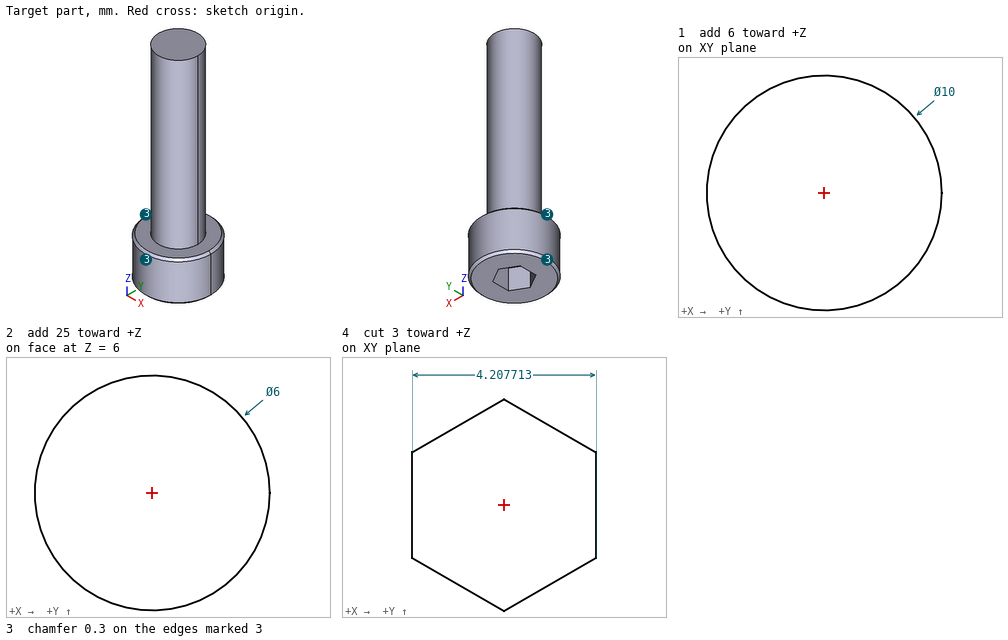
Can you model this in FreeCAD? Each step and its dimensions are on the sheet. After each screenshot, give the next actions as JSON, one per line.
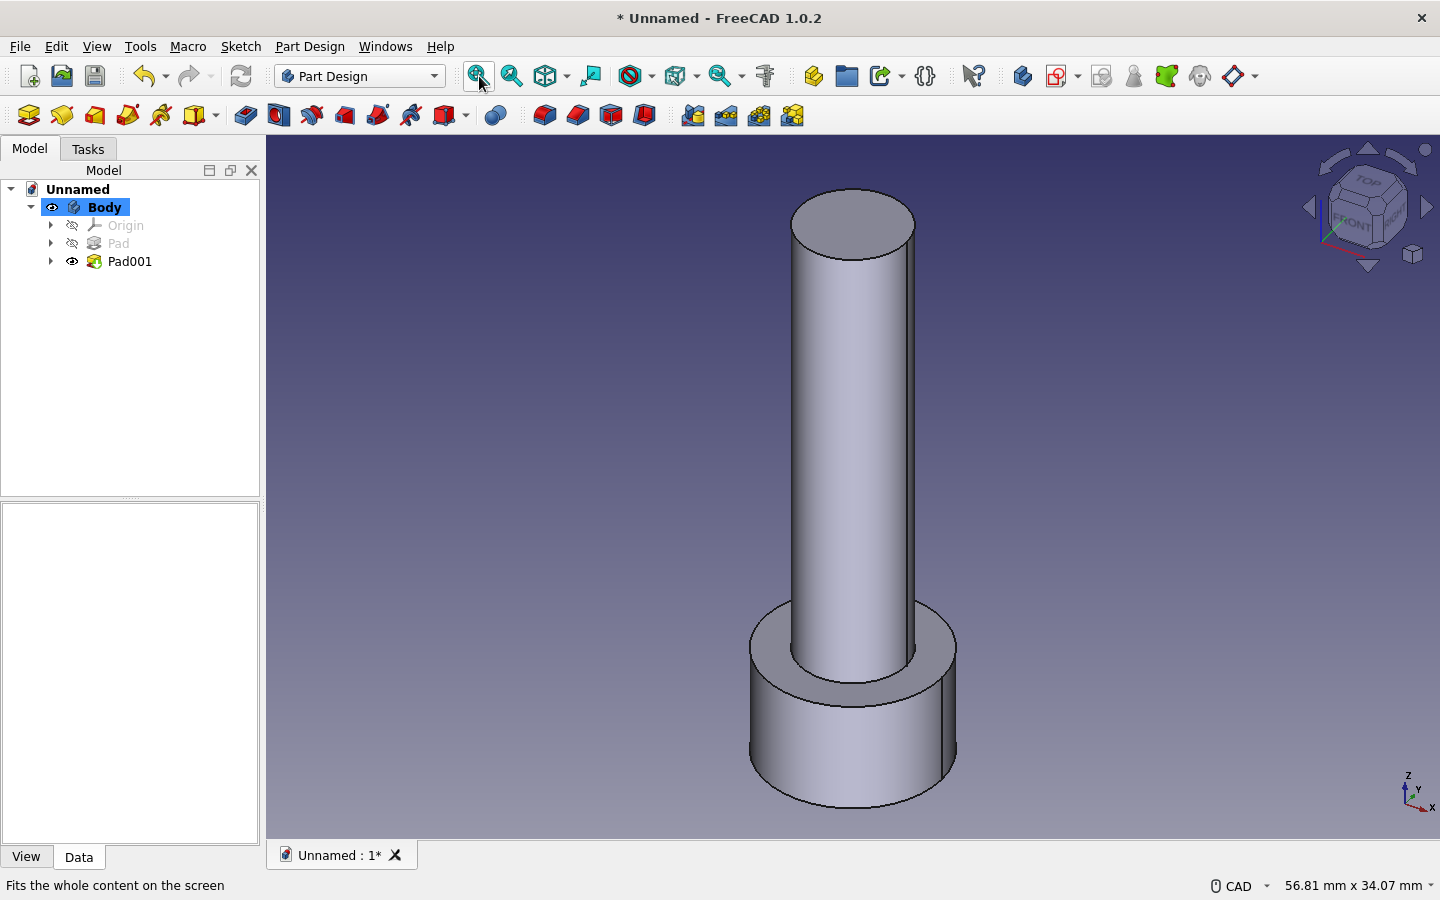
{"action": "left_click", "coordinate": [750, 653]}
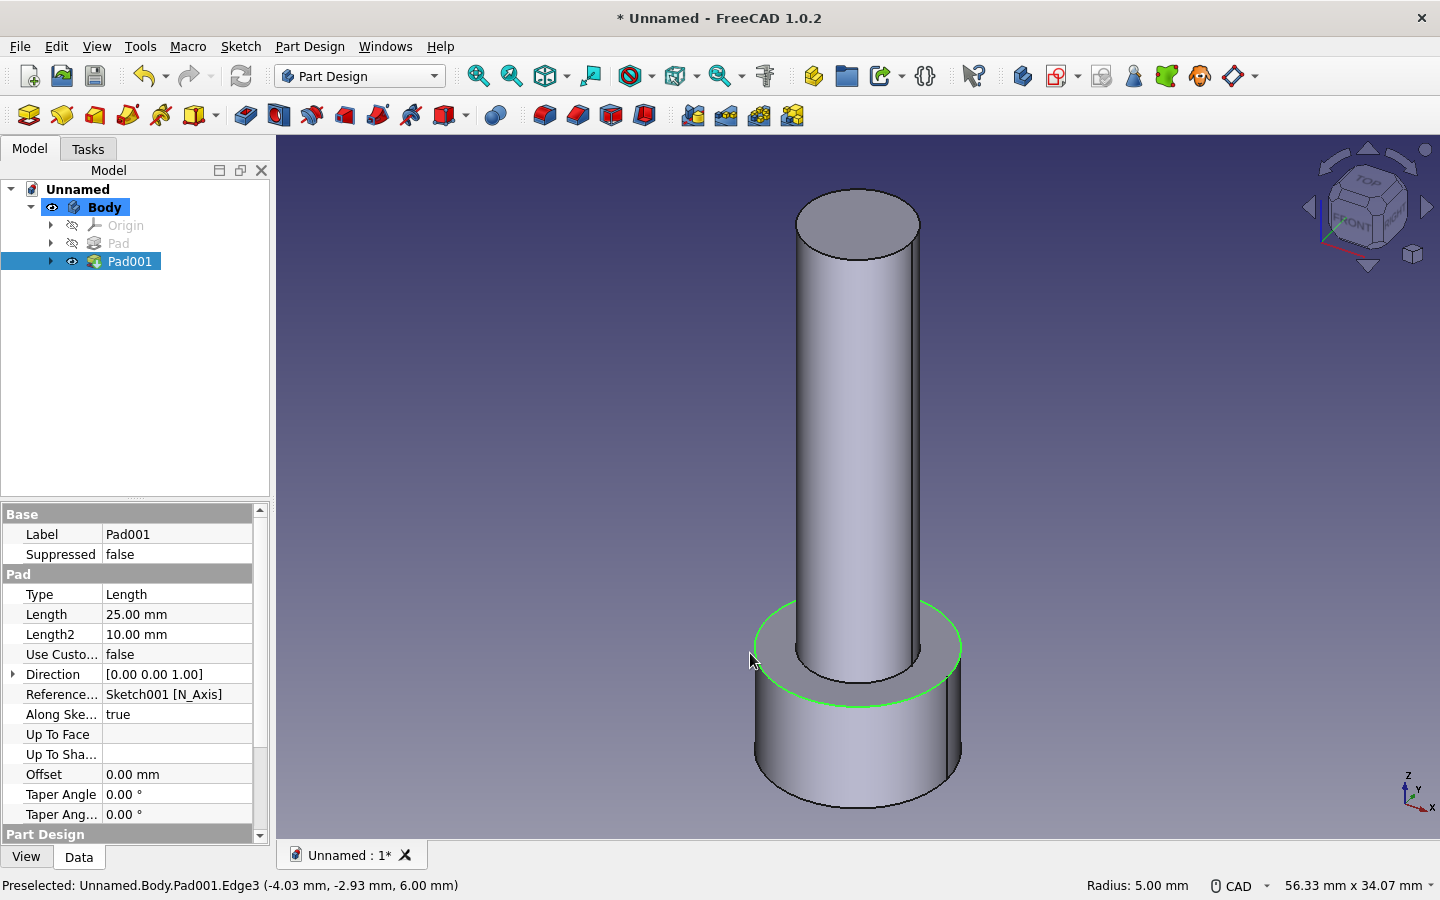
{"action": "key", "text": "0"}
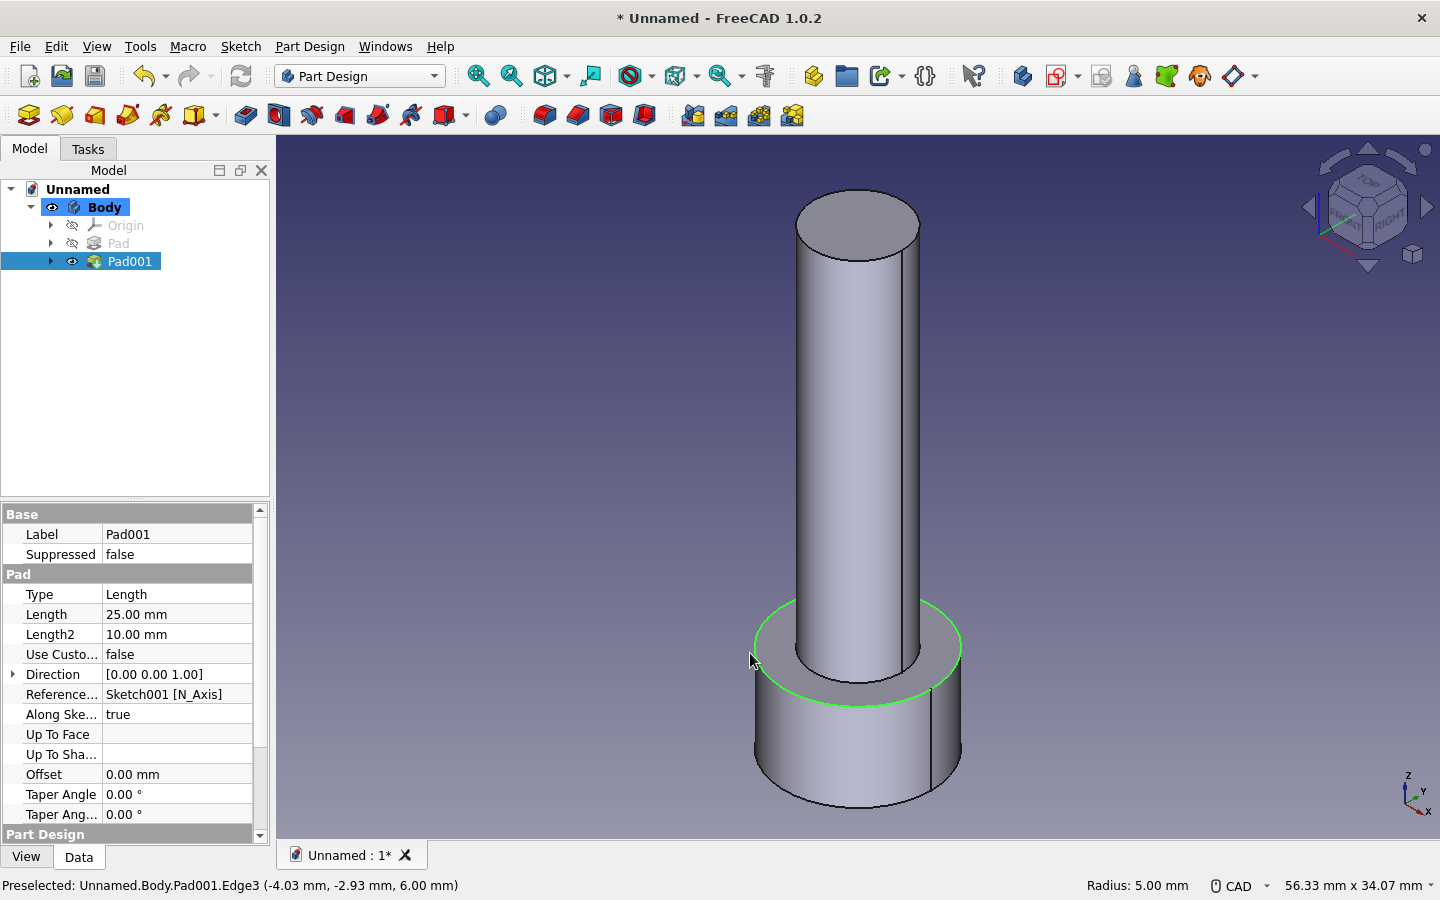
{"action": "key", "text": "2"}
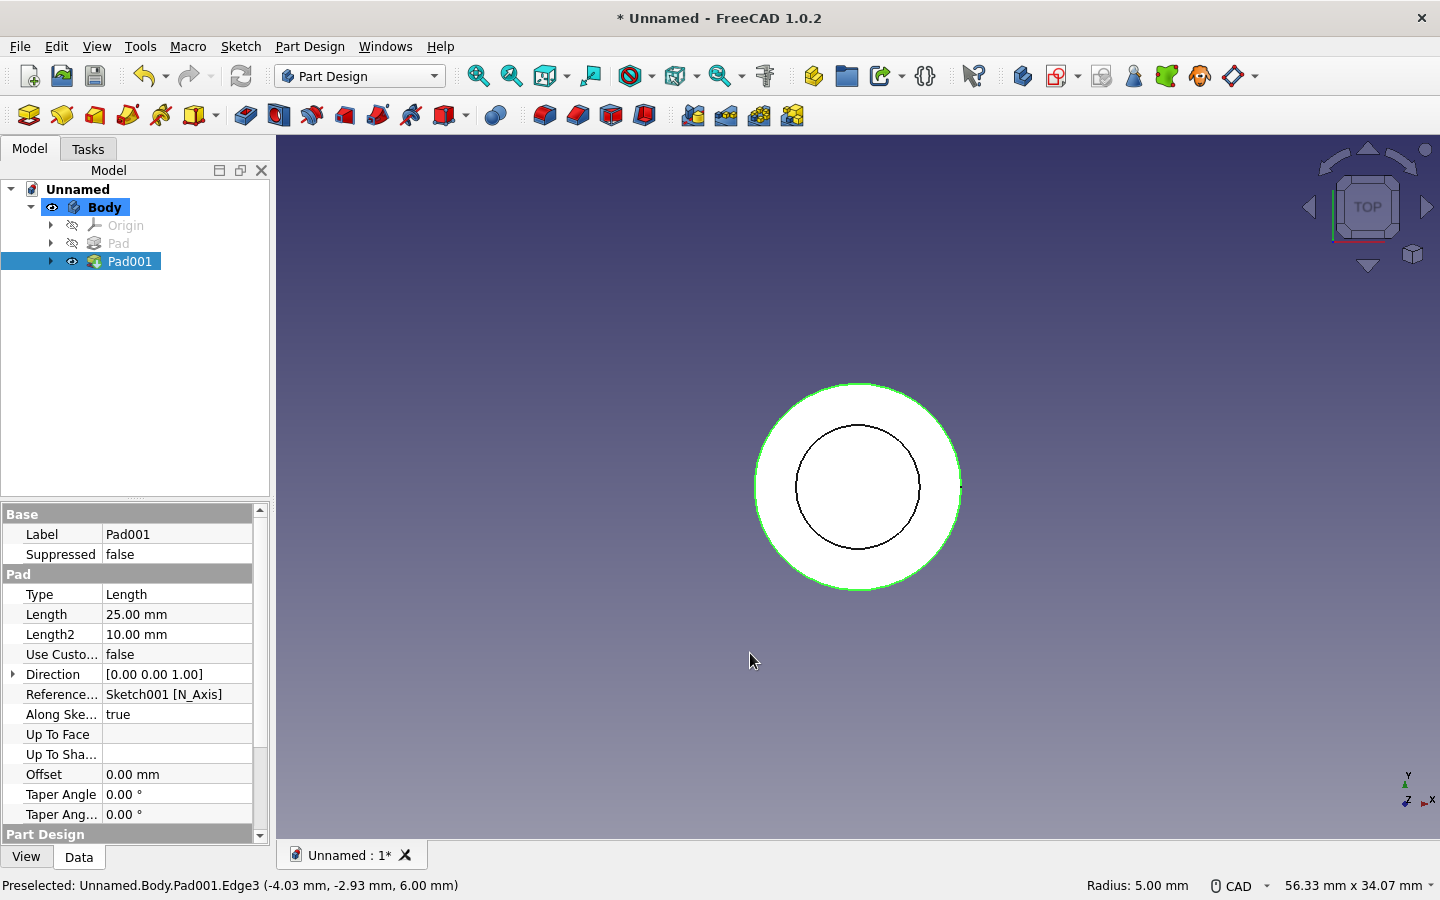
{"action": "left_click", "coordinate": [479, 76]}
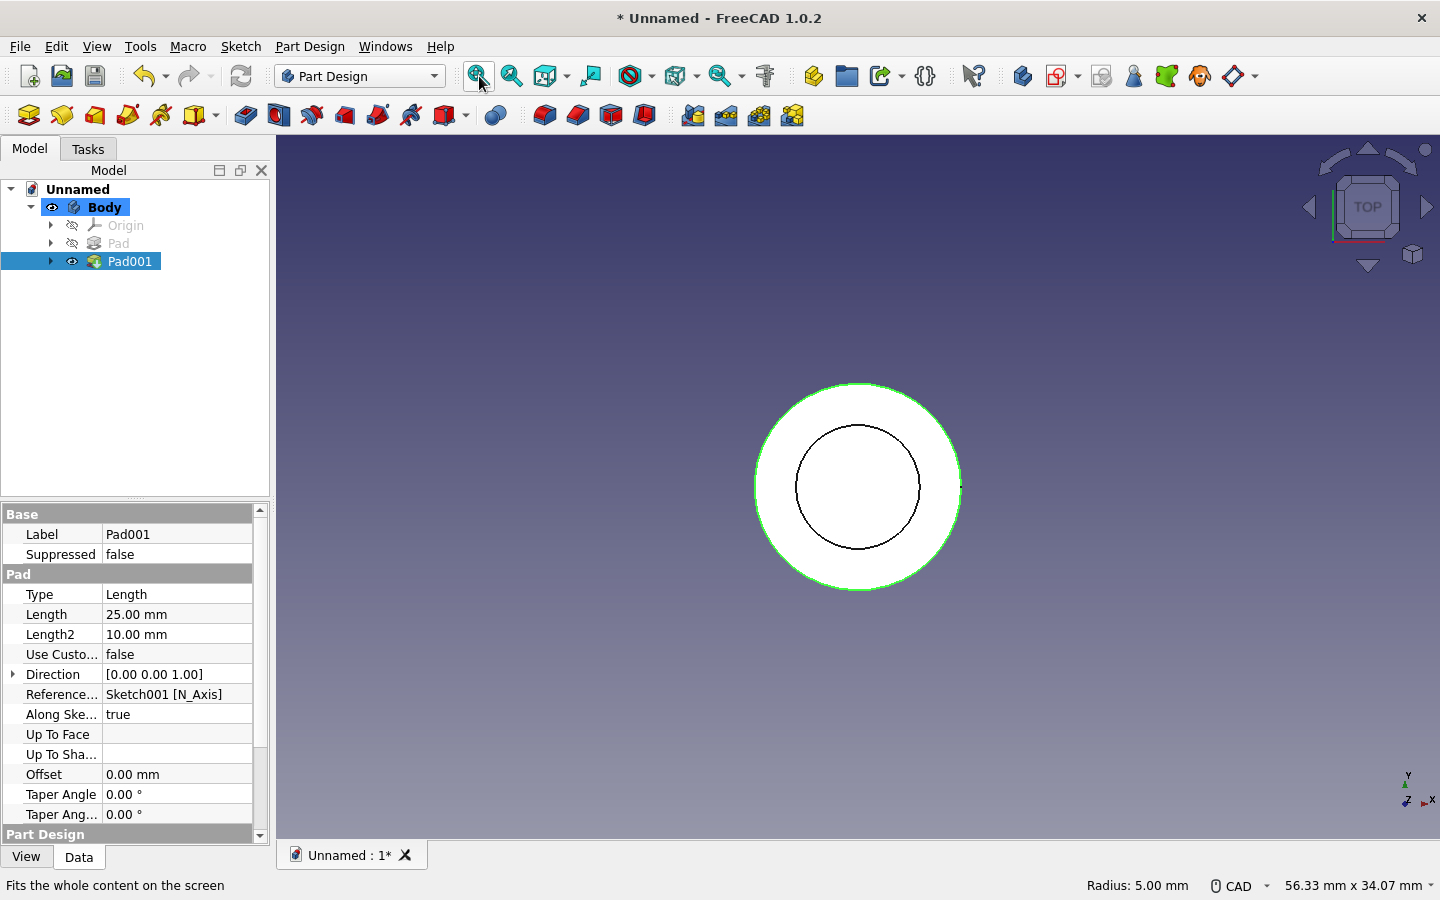
{"action": "key", "text": "1"}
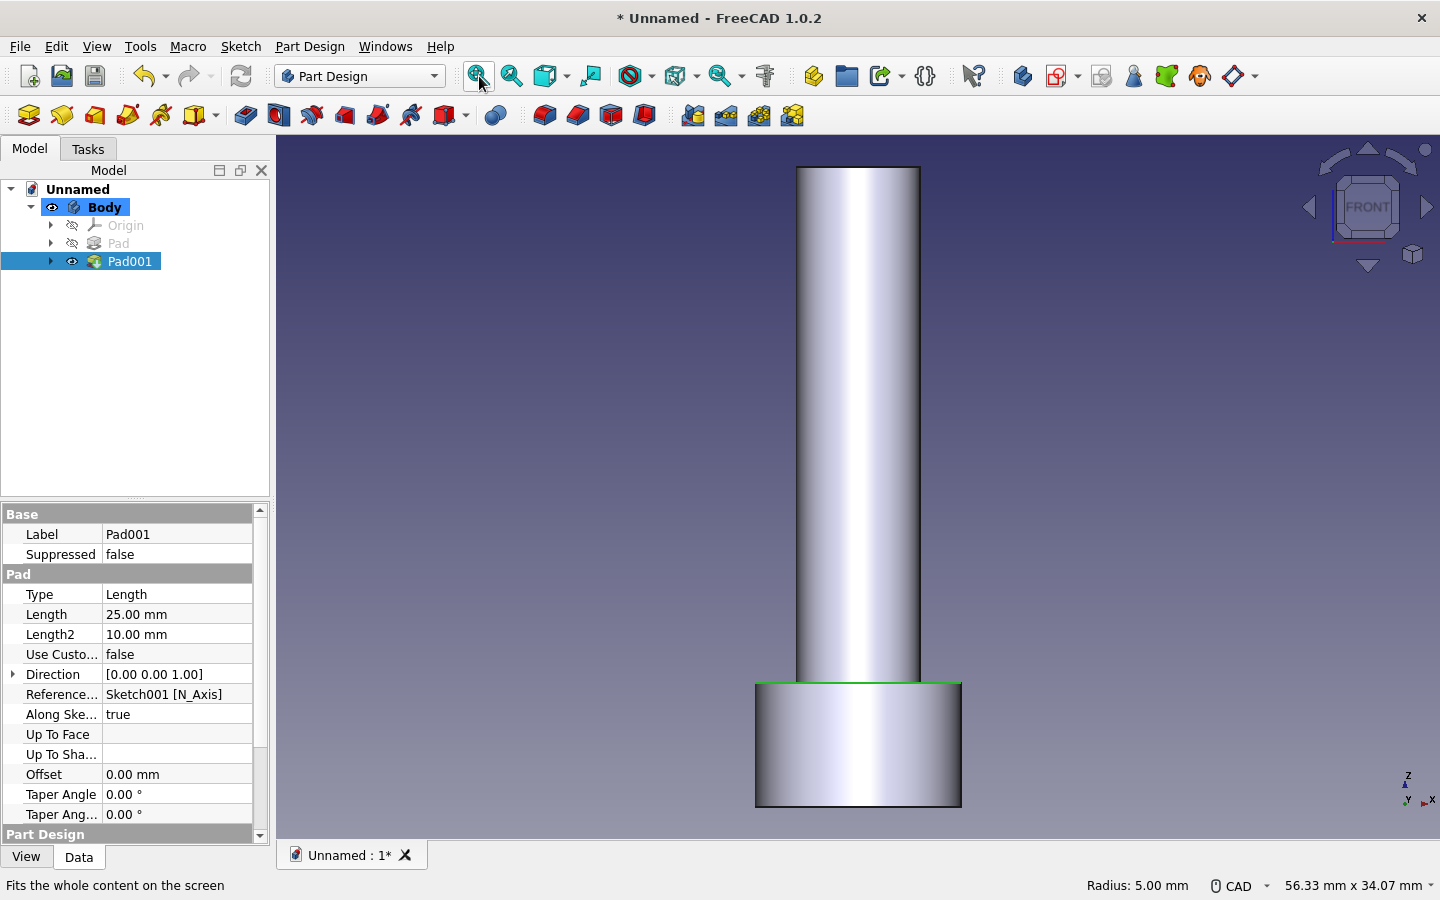
{"action": "left_click", "coordinate": [774, 806], "text": "ctrl"}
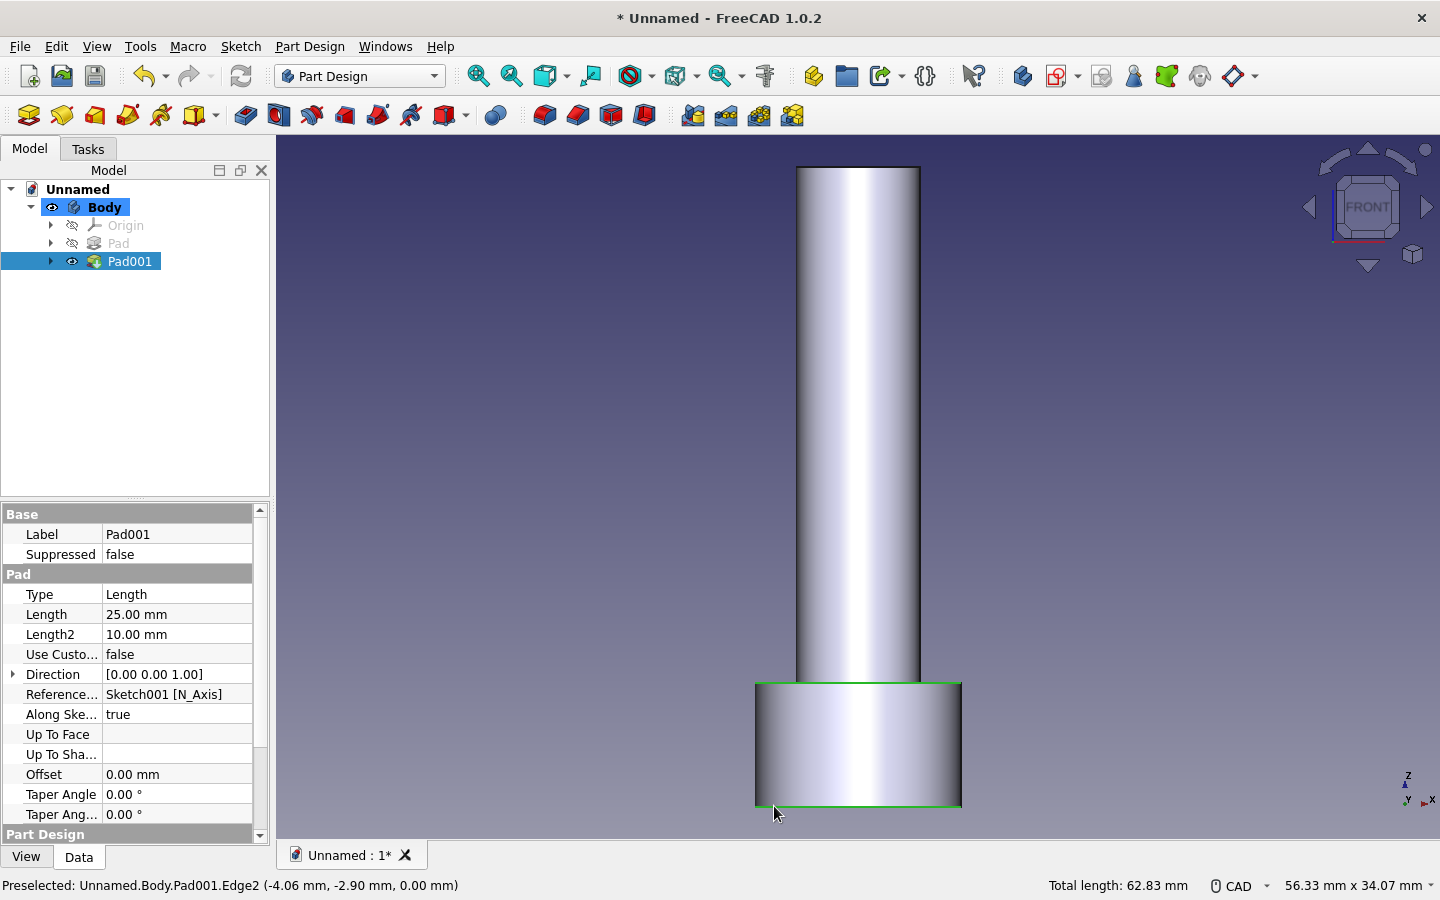
{"action": "left_click", "coordinate": [578, 116]}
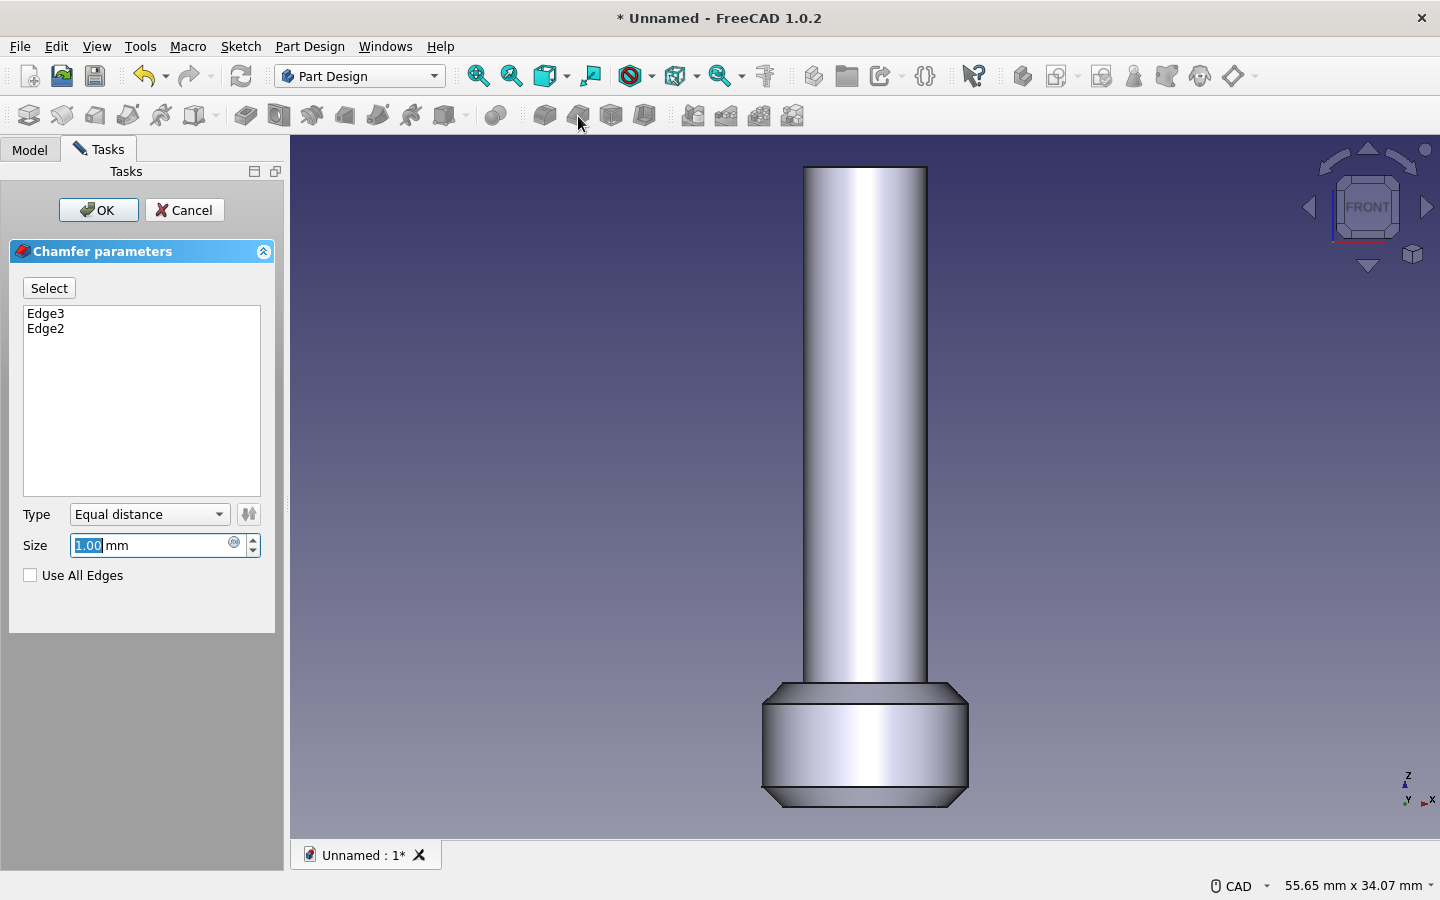
{"action": "type", "text": "0.3"}
{"action": "key", "text": "Tab"}